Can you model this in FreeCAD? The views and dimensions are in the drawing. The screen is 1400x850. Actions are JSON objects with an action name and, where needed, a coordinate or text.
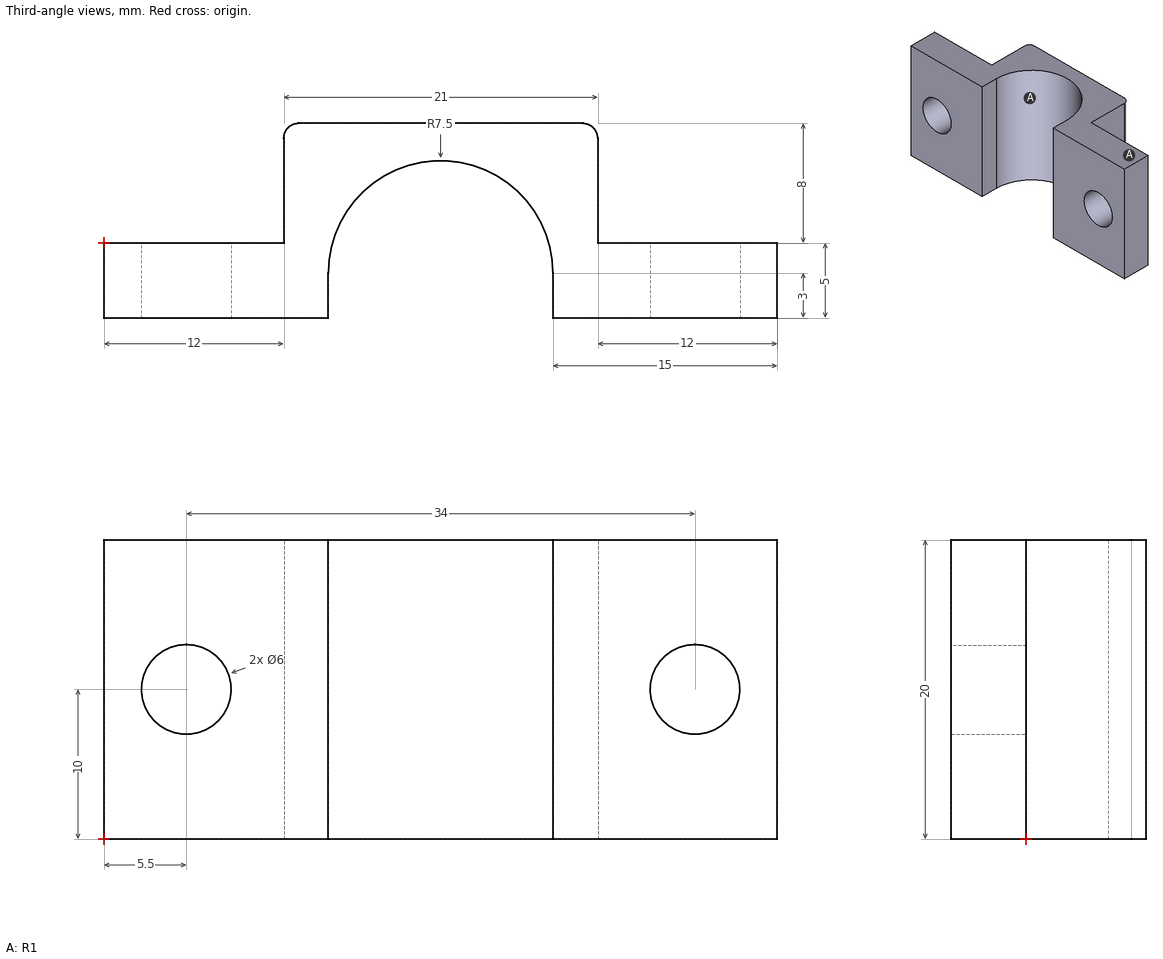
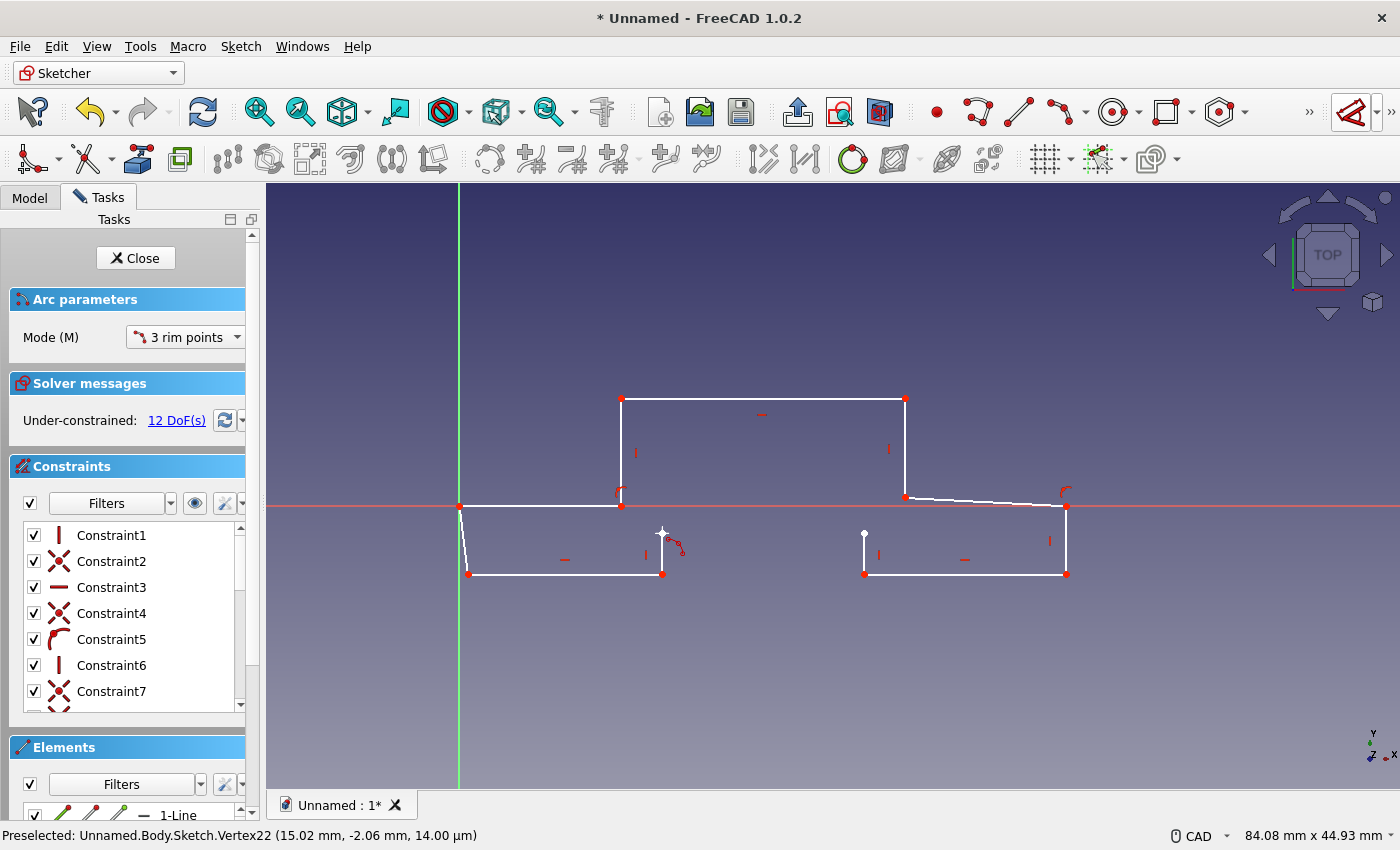
{"action": "left_click", "coordinate": [662, 534]}
{"action": "left_click", "coordinate": [864, 534]}
{"action": "left_click", "coordinate": [763, 432]}
{"action": "key", "text": "Escape"}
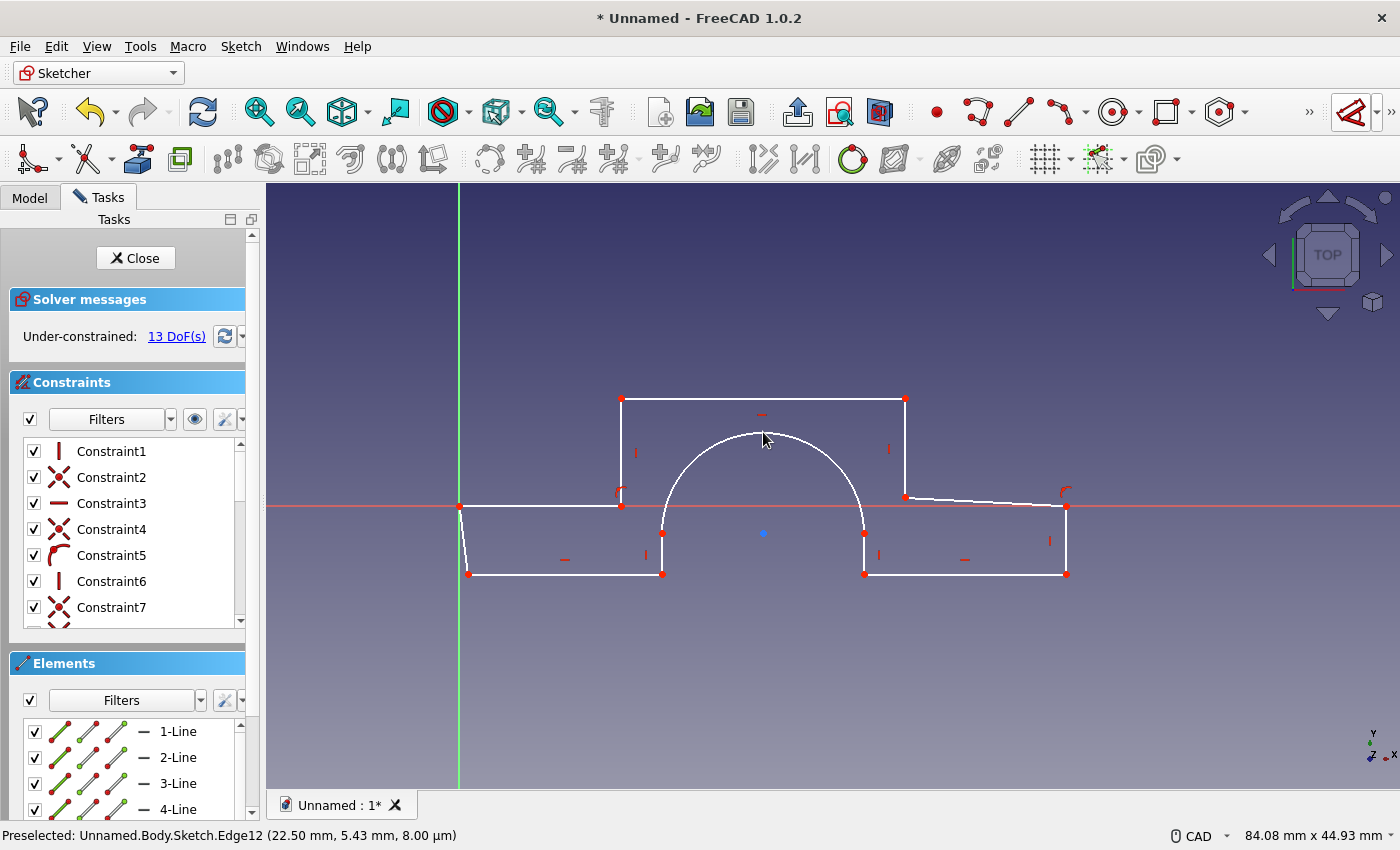
{"action": "left_click", "coordinate": [864, 546]}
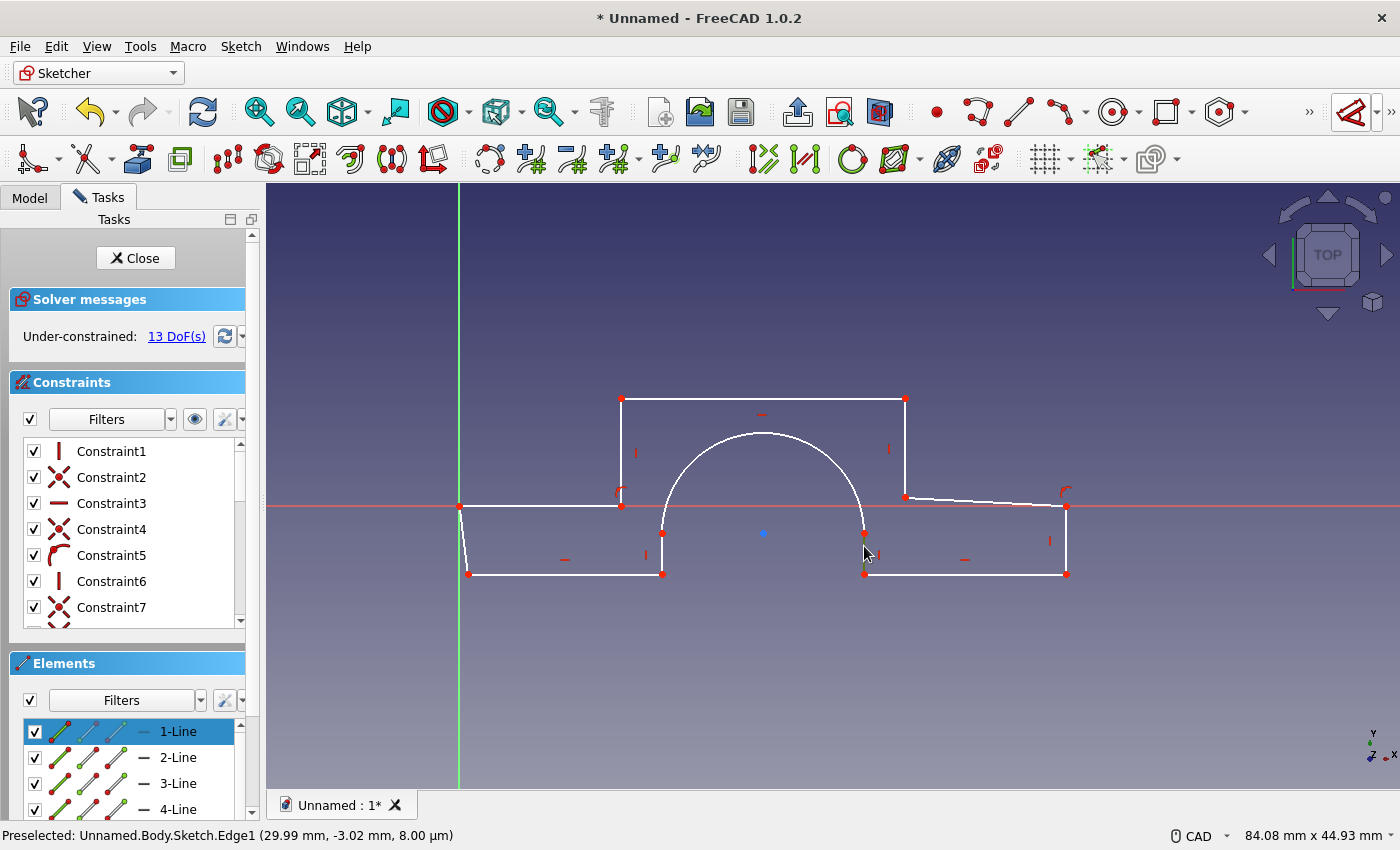
{"action": "left_click", "coordinate": [822, 452]}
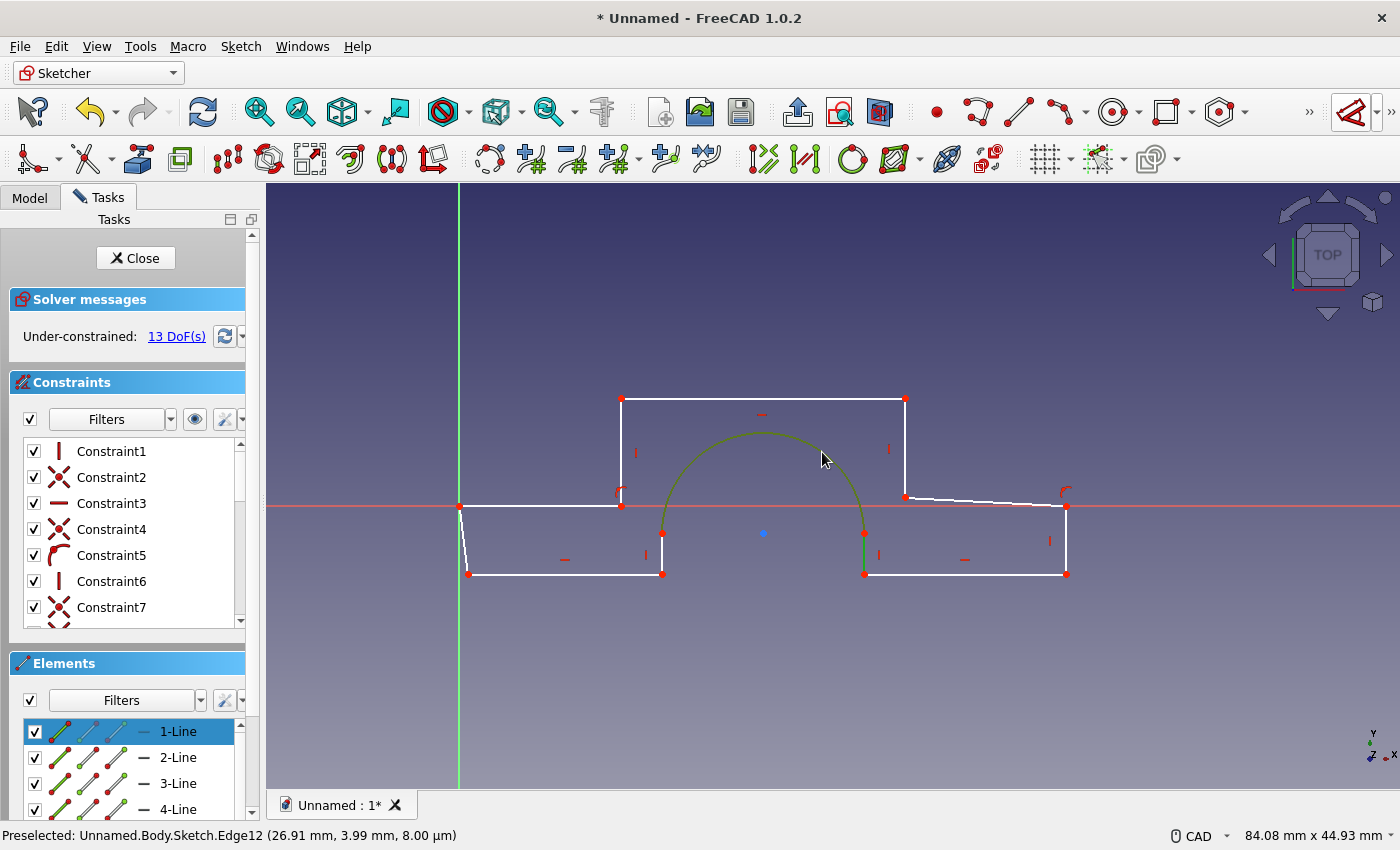
{"action": "key", "text": "t"}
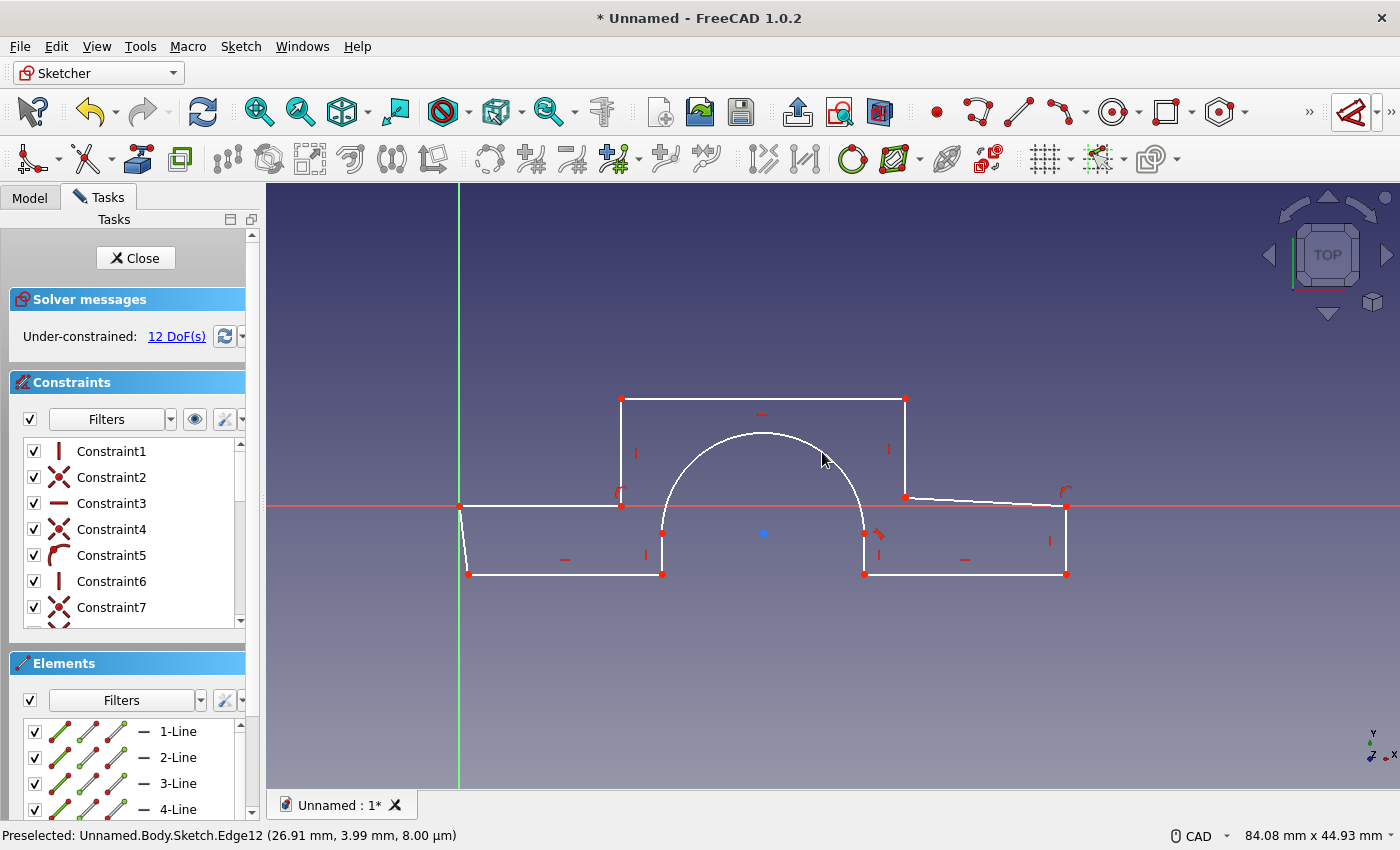
{"action": "left_click", "coordinate": [662, 563]}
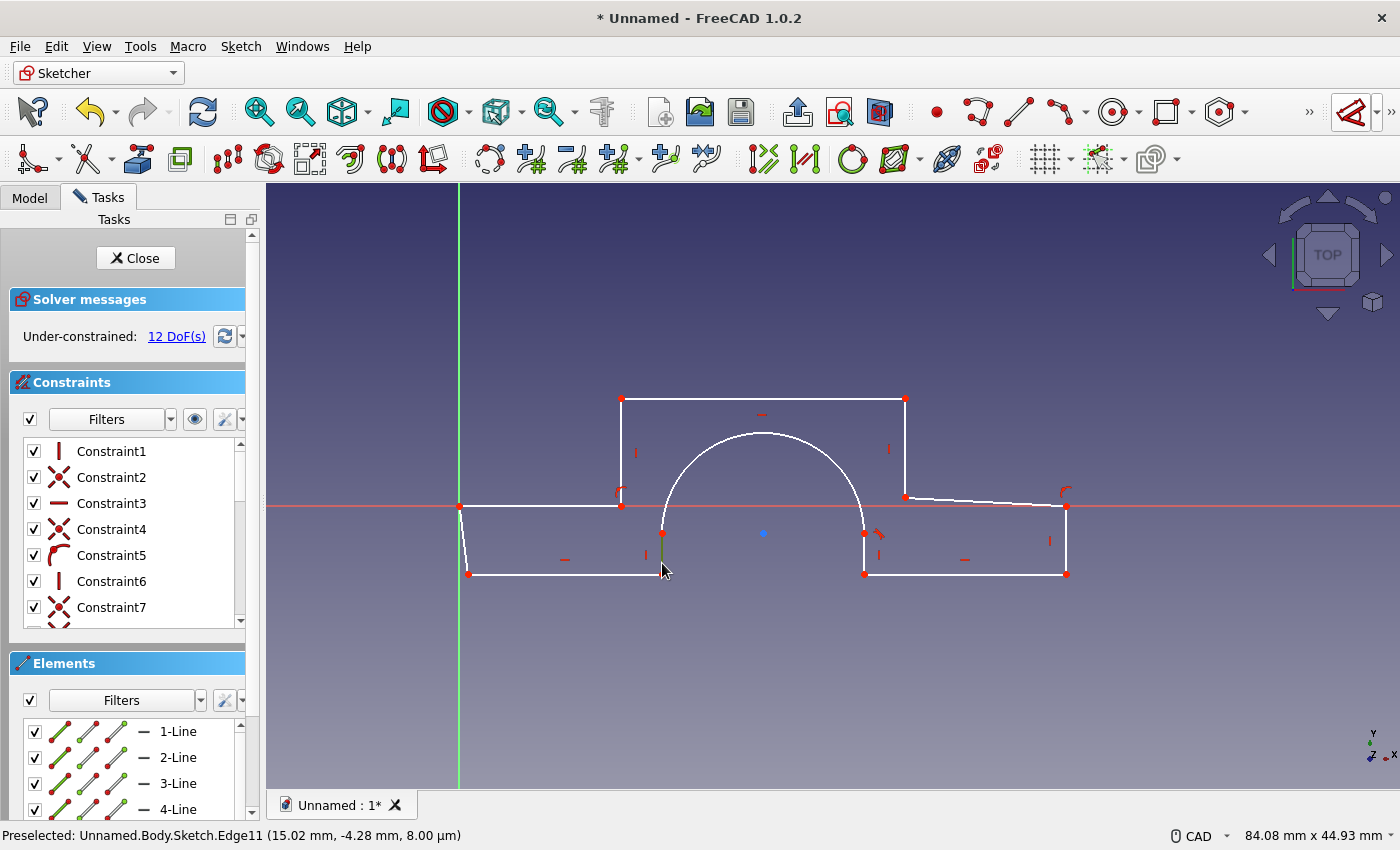
{"action": "left_click", "coordinate": [822, 452]}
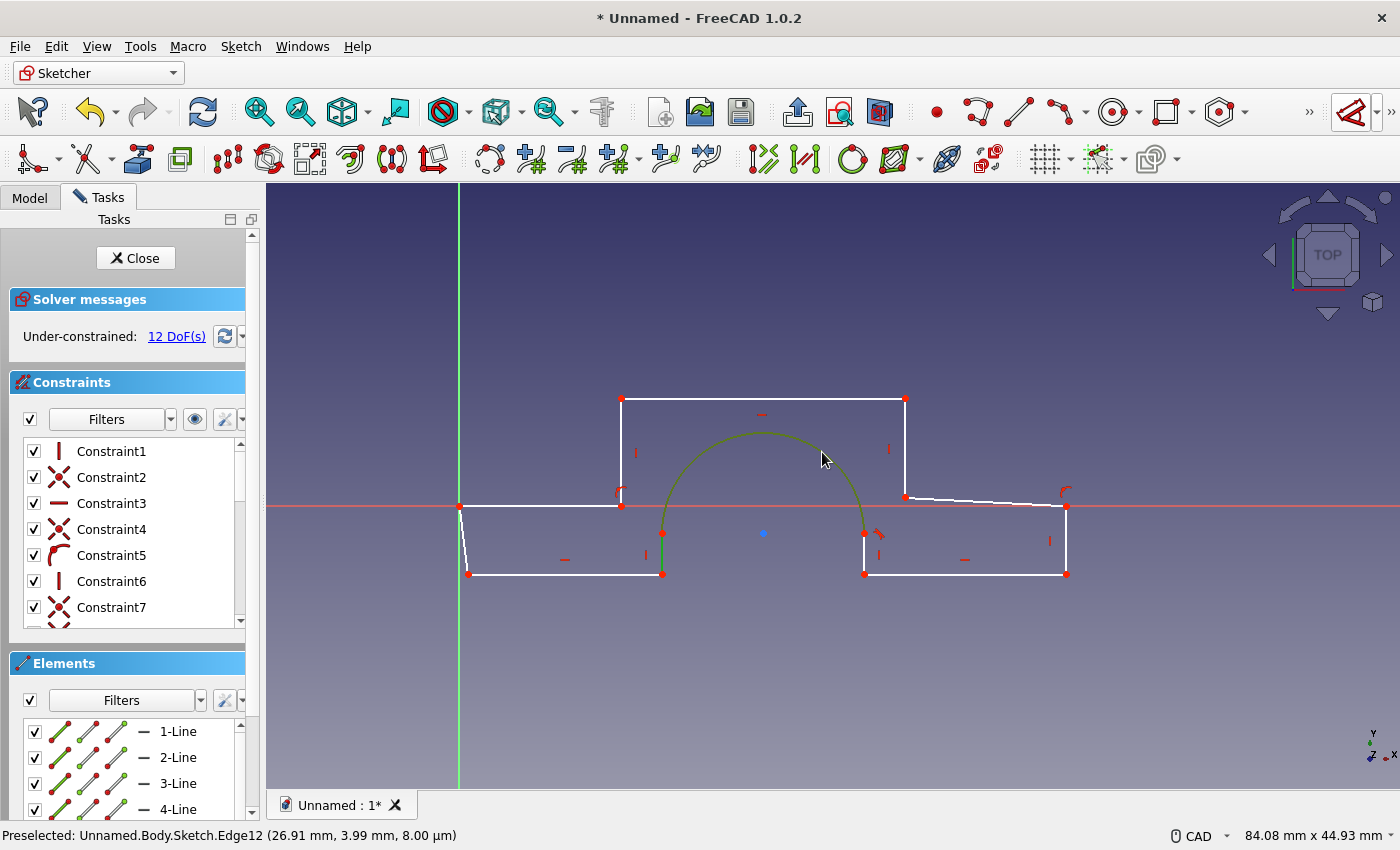
{"action": "key", "text": "t"}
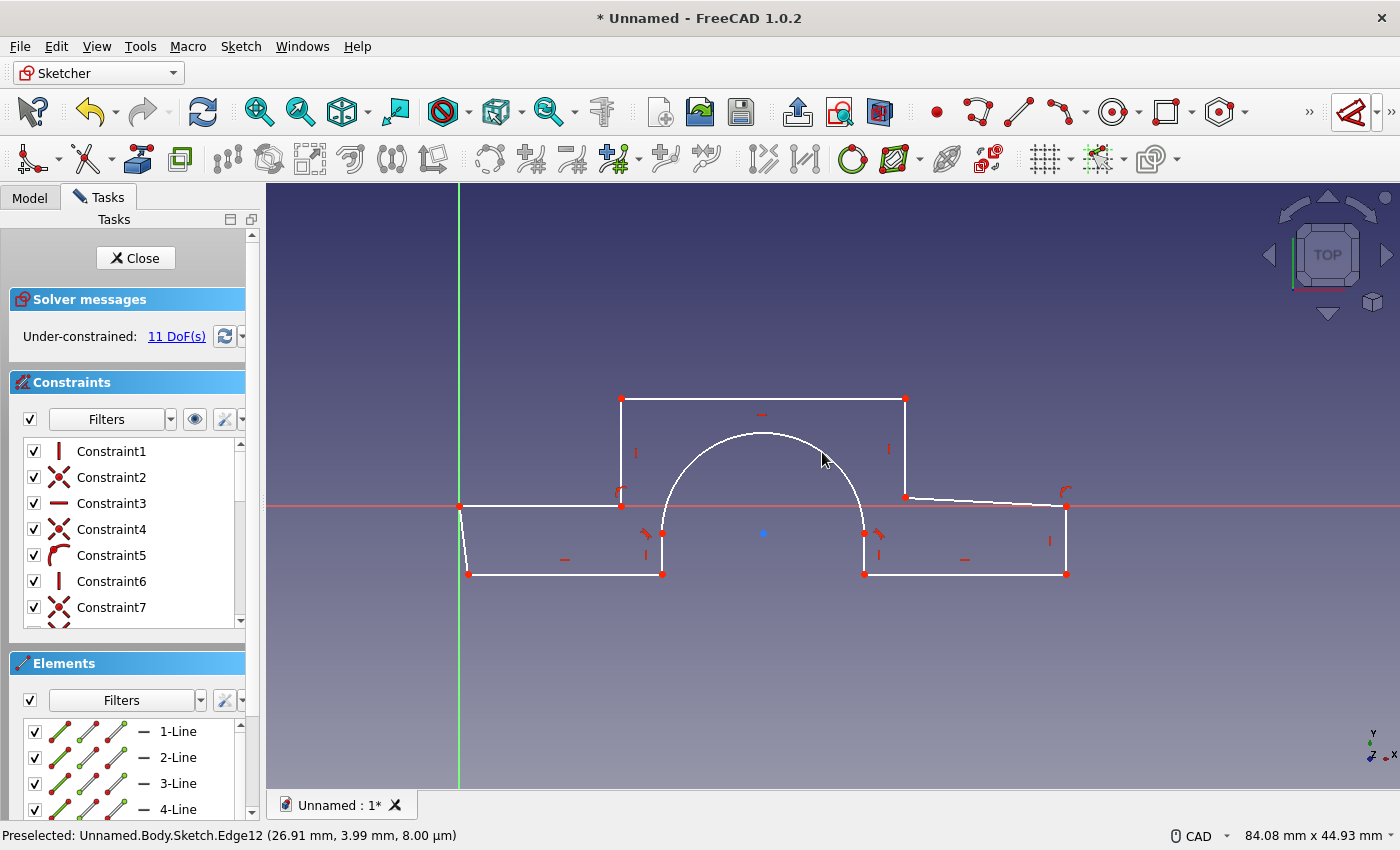
{"action": "left_click", "coordinate": [1018, 504]}